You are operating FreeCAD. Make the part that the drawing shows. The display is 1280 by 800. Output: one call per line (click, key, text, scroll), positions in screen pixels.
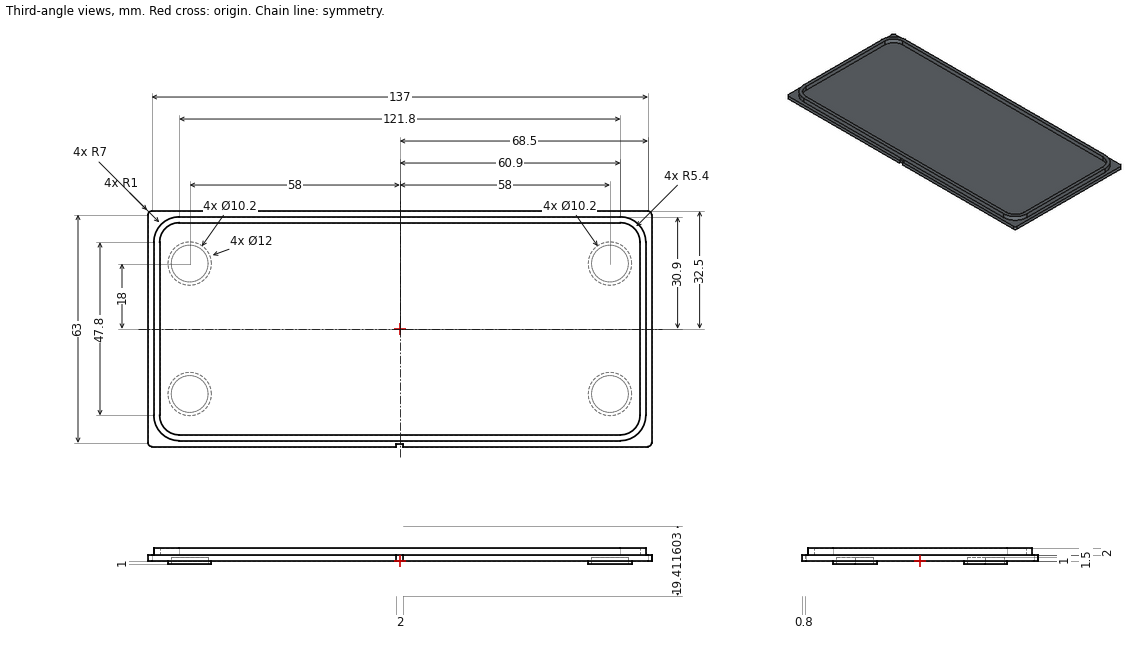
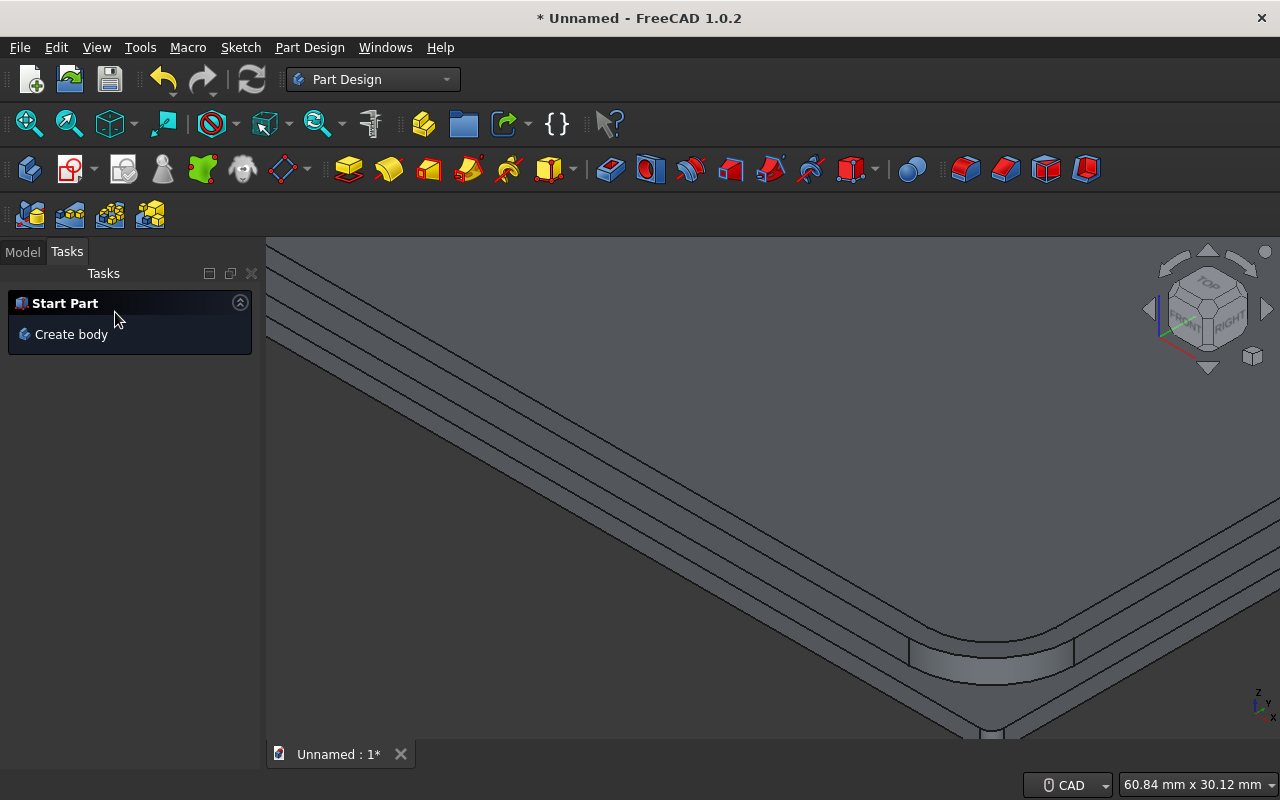
click(30, 124)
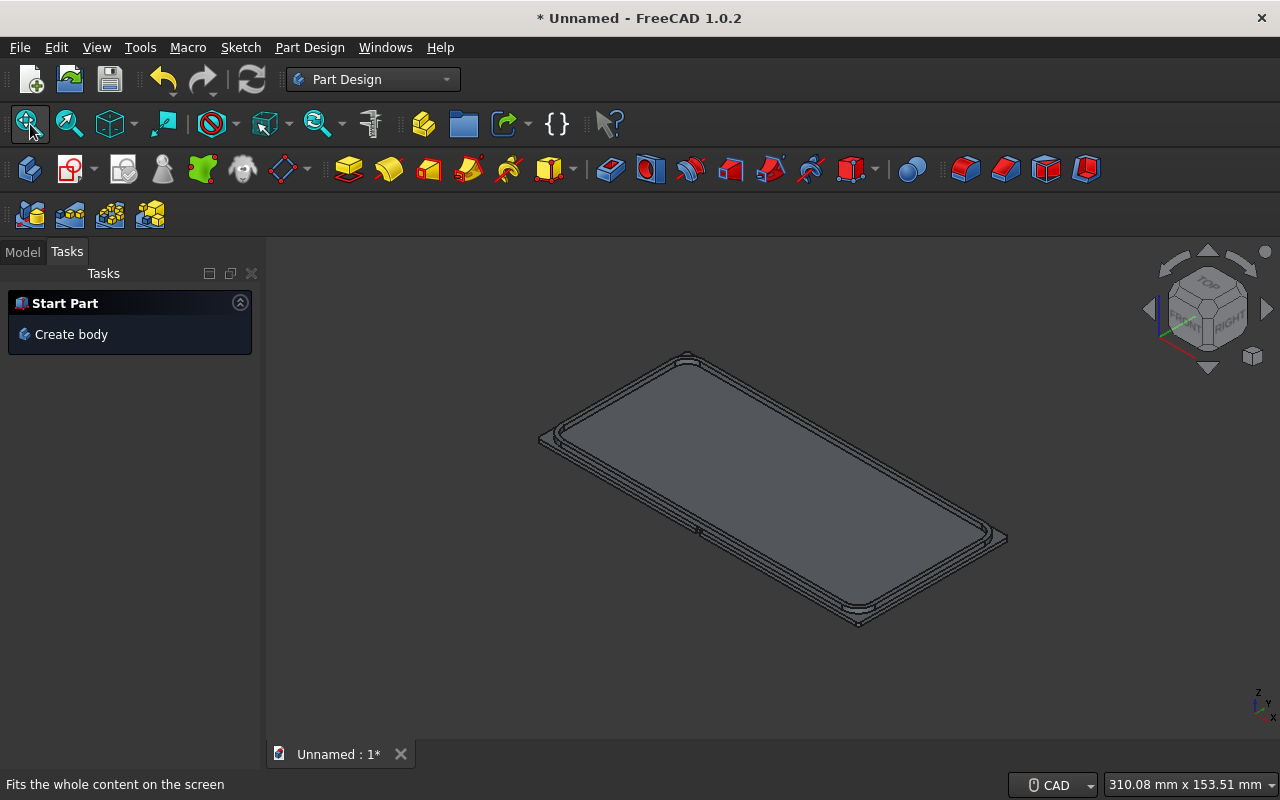
click(23, 251)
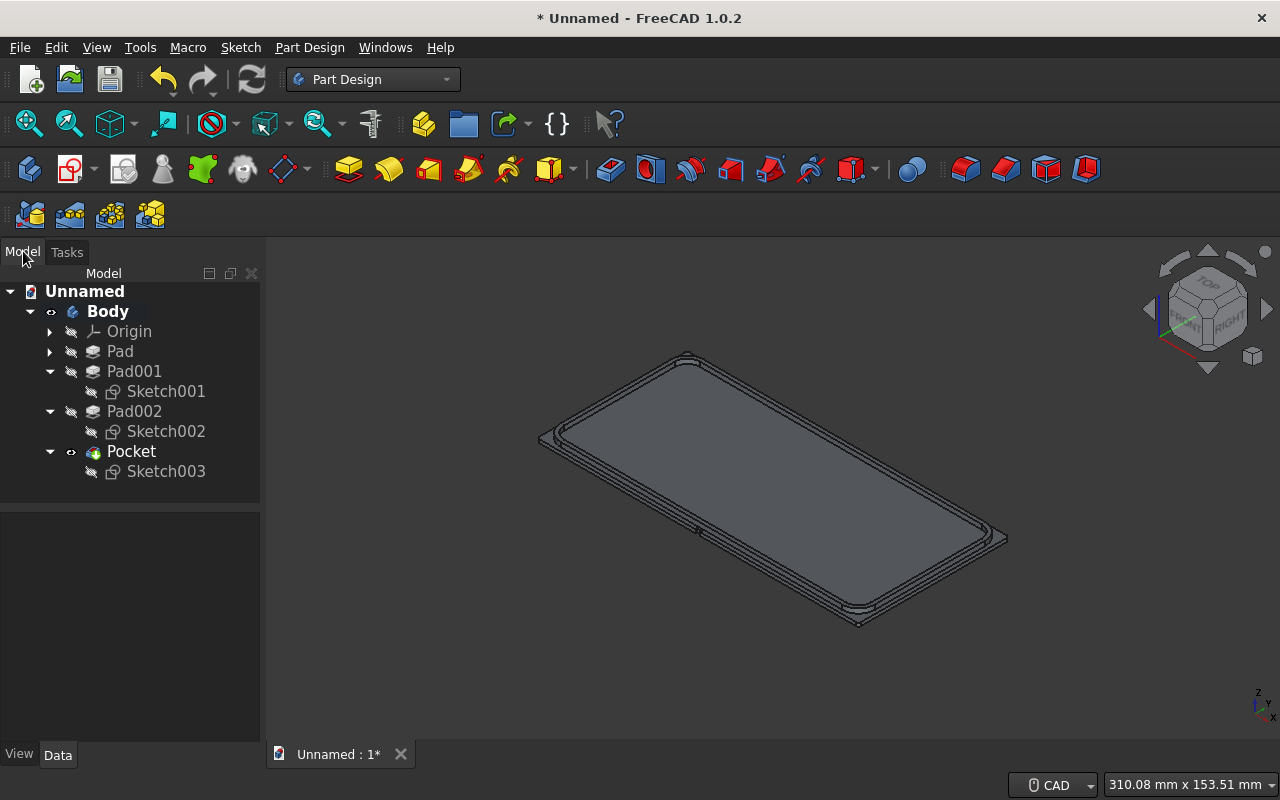
click(50, 332)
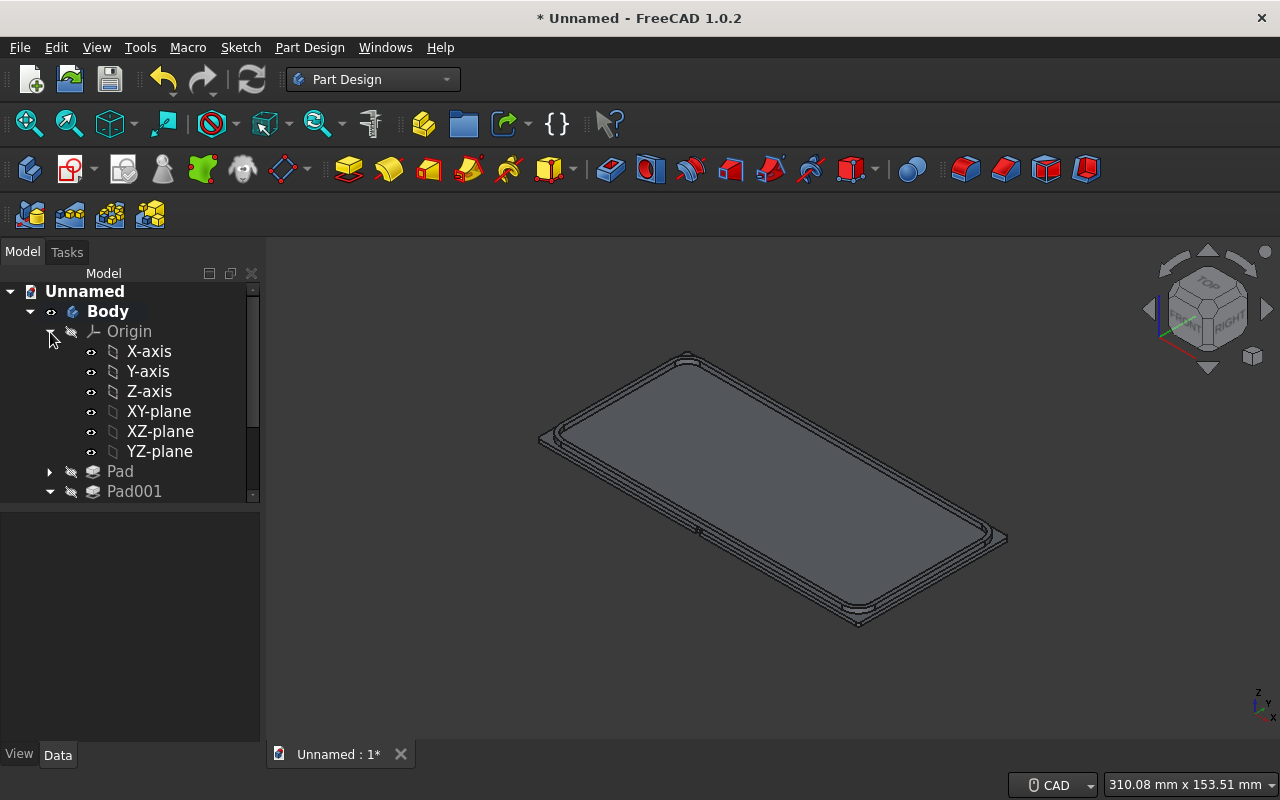
click(136, 412)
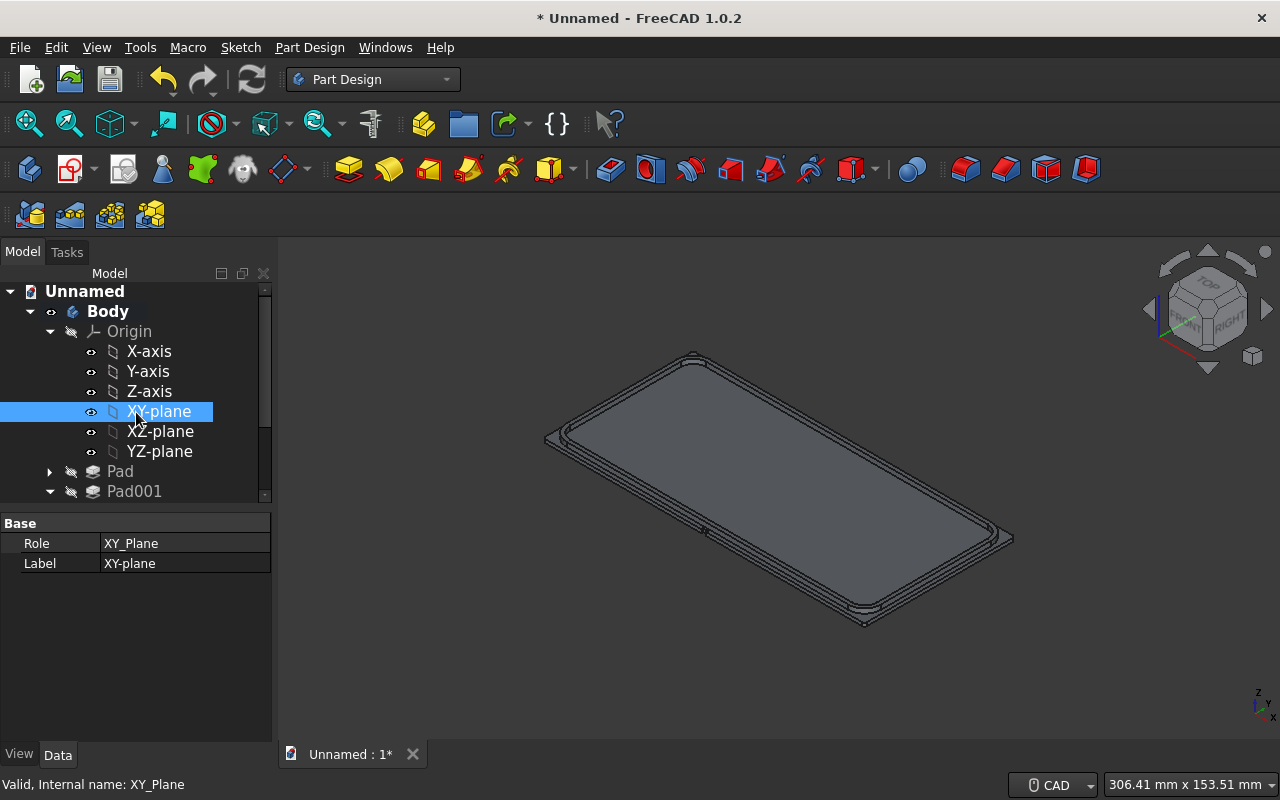
click(284, 170)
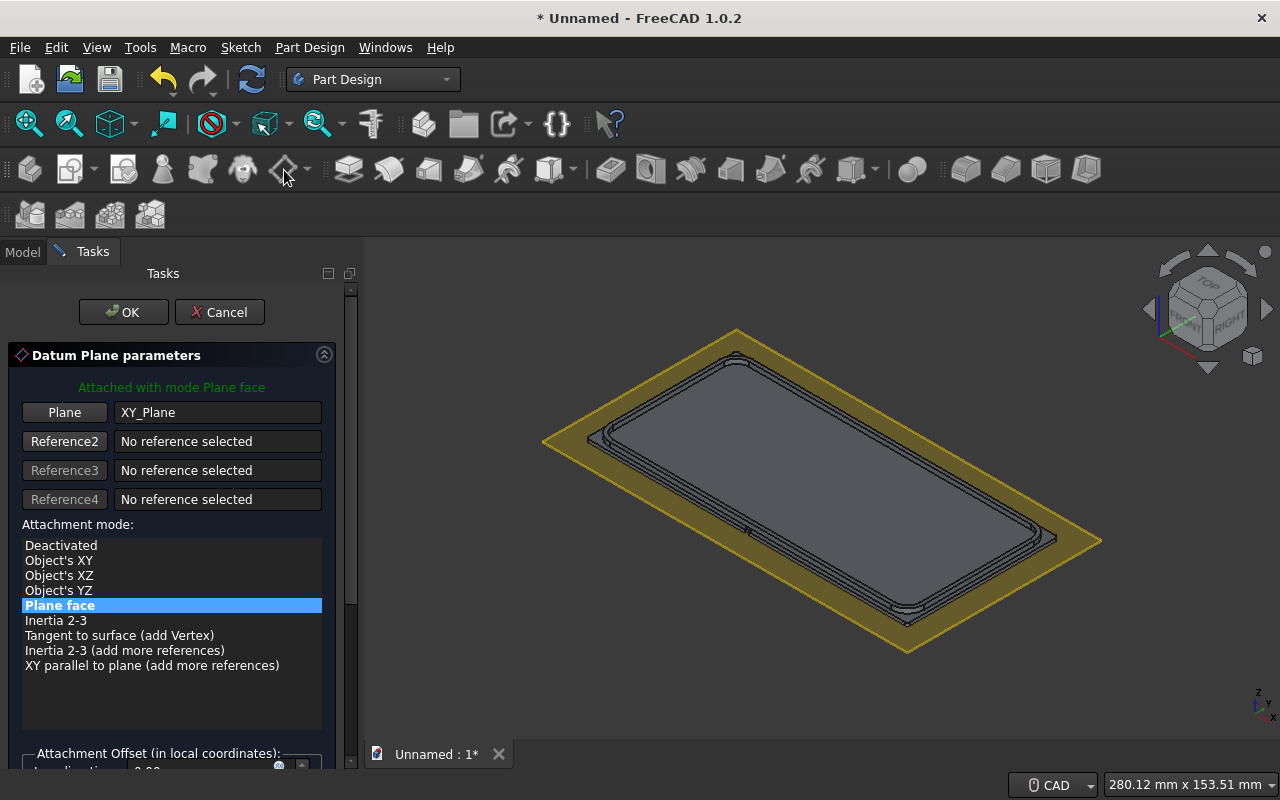
scroll(351, 526, down, 3)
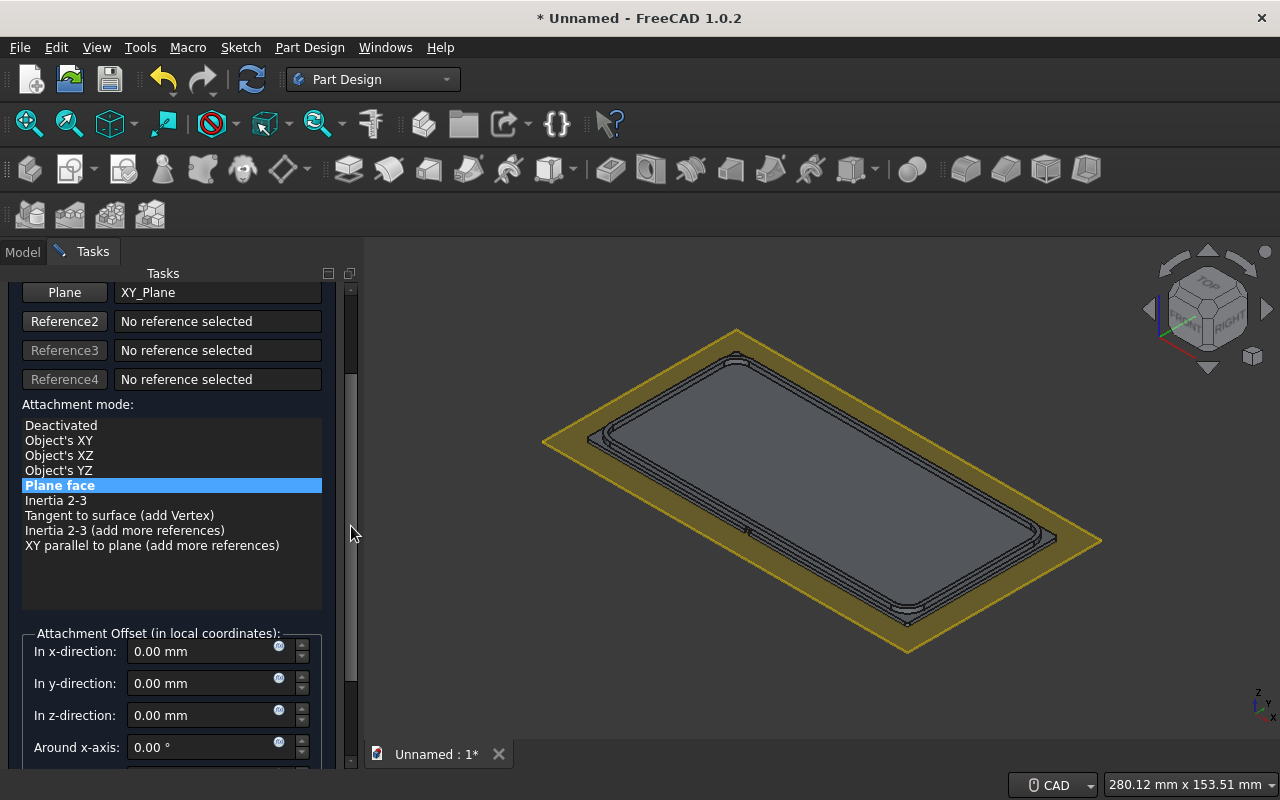
triple_click(210, 655)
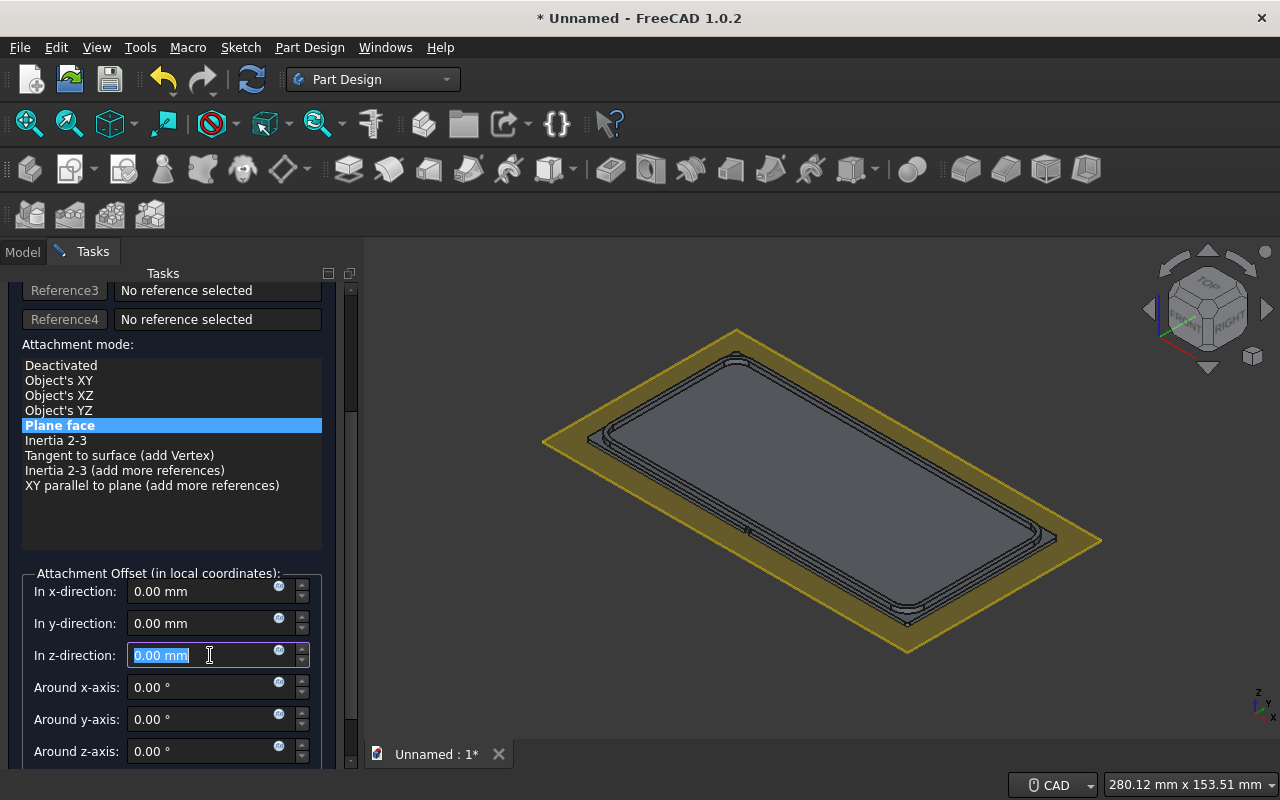
text(1)
key(Tab)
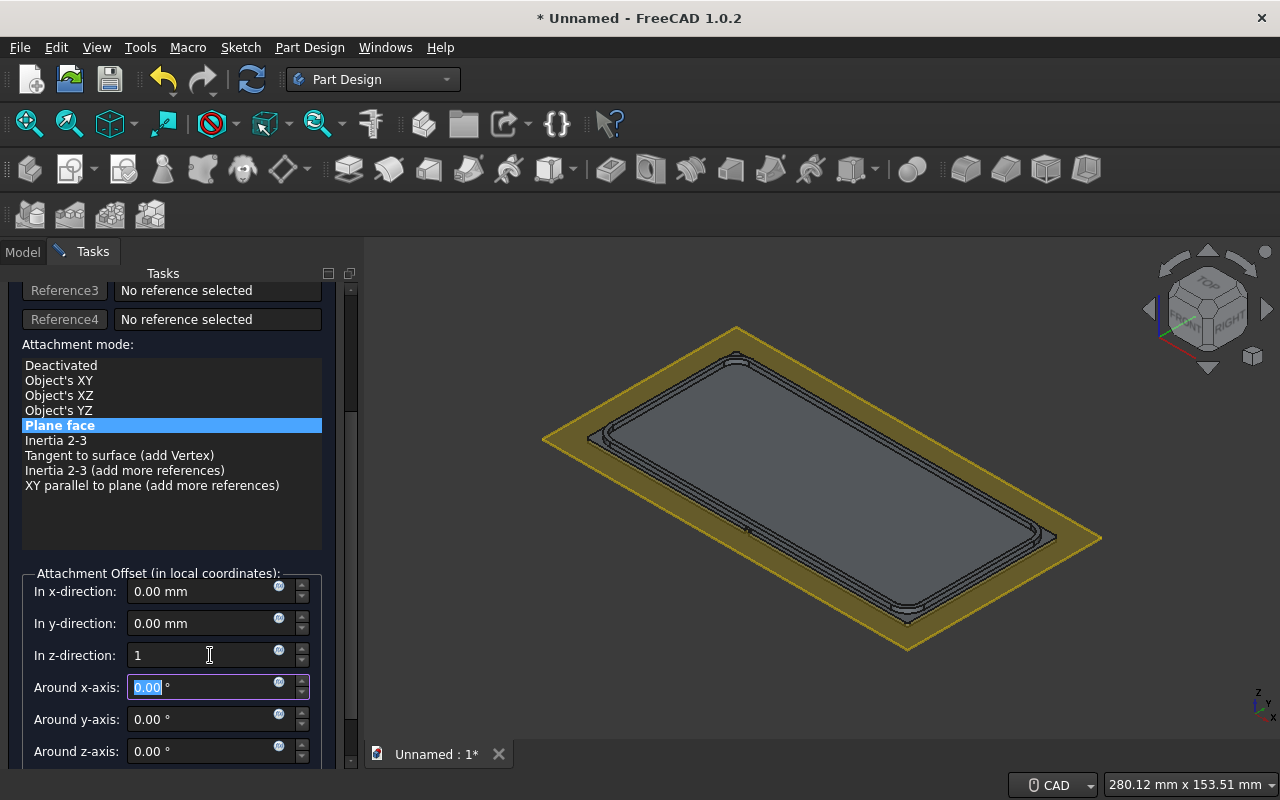
scroll(351, 526, up, 4)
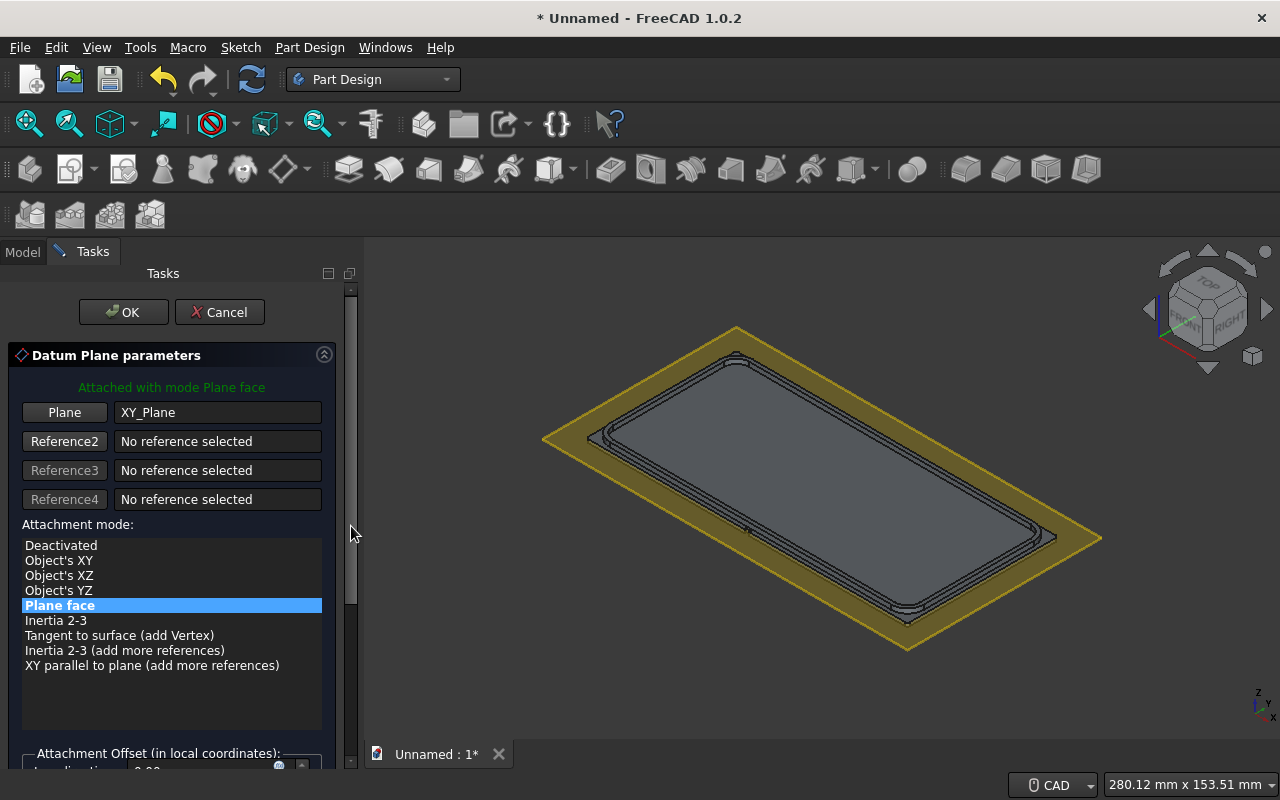
click(124, 312)